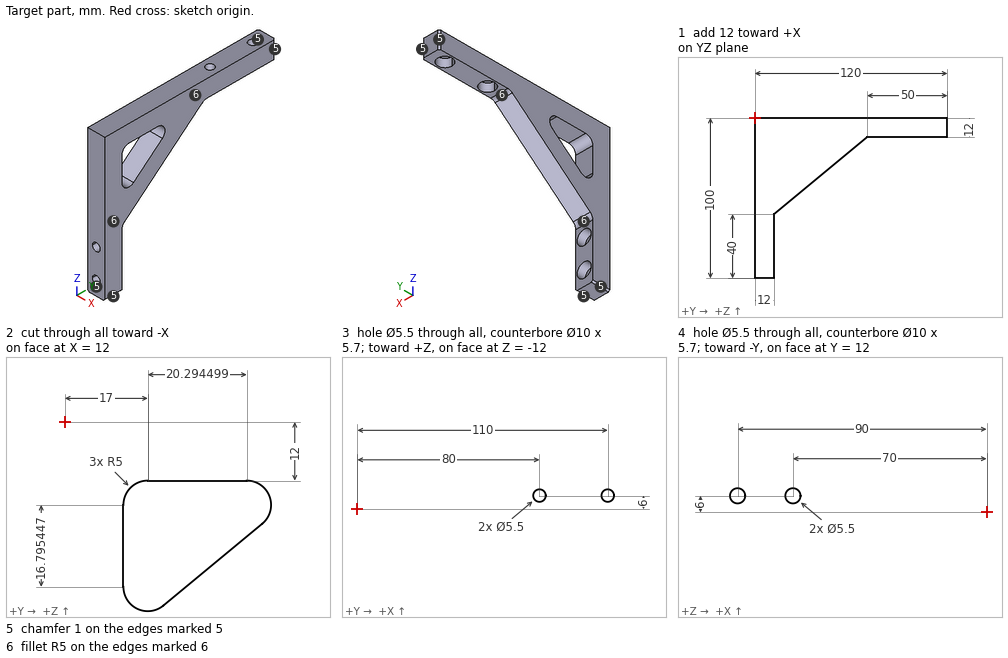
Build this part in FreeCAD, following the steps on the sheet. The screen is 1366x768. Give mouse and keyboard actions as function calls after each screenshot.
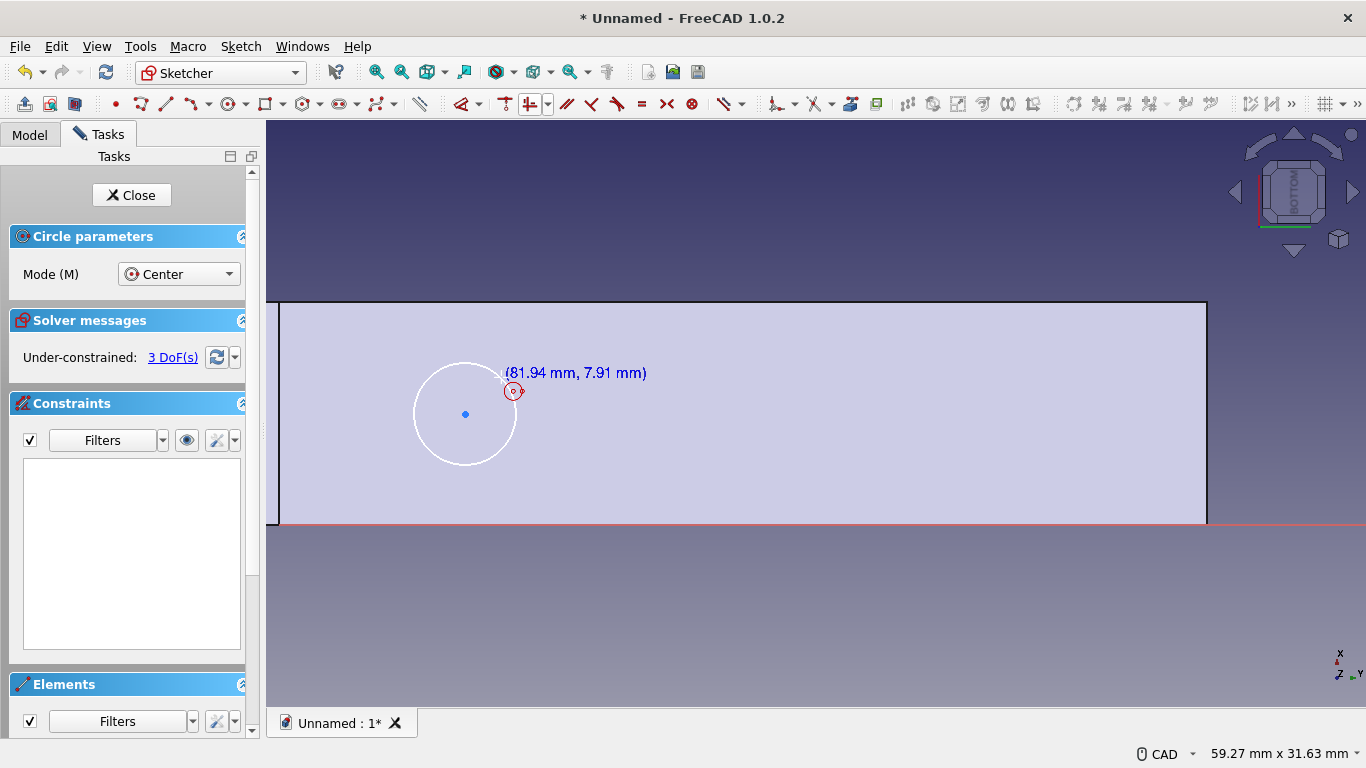
click(1022, 413)
click(1058, 377)
key(Escape)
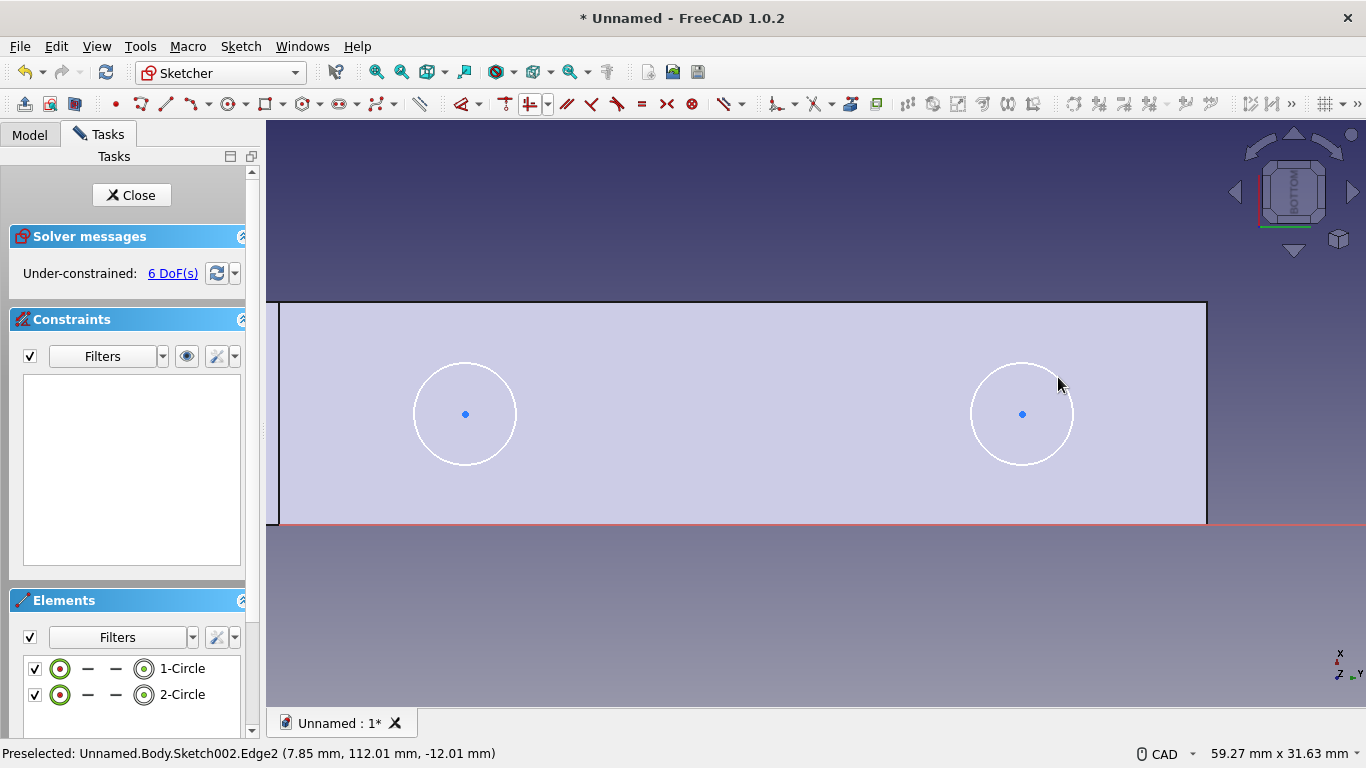
click(501, 378)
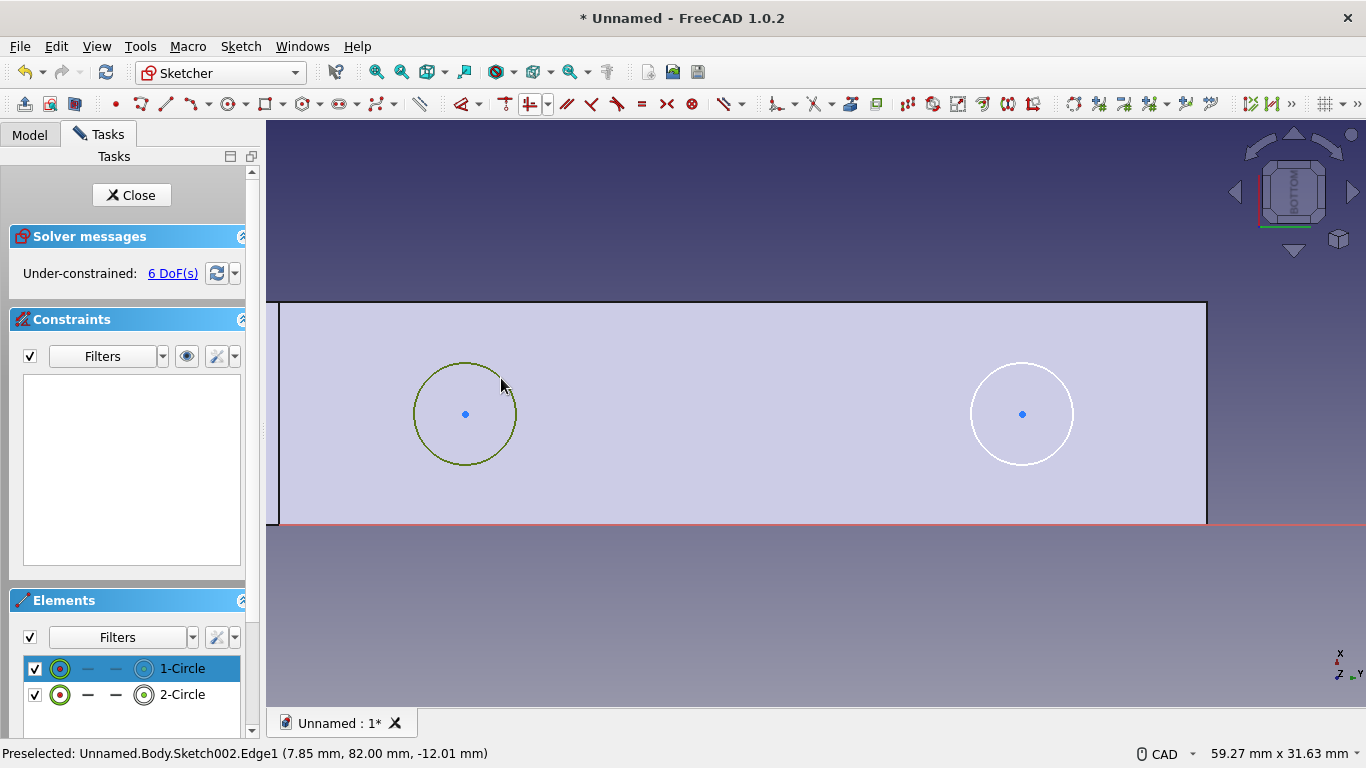
click(1058, 378)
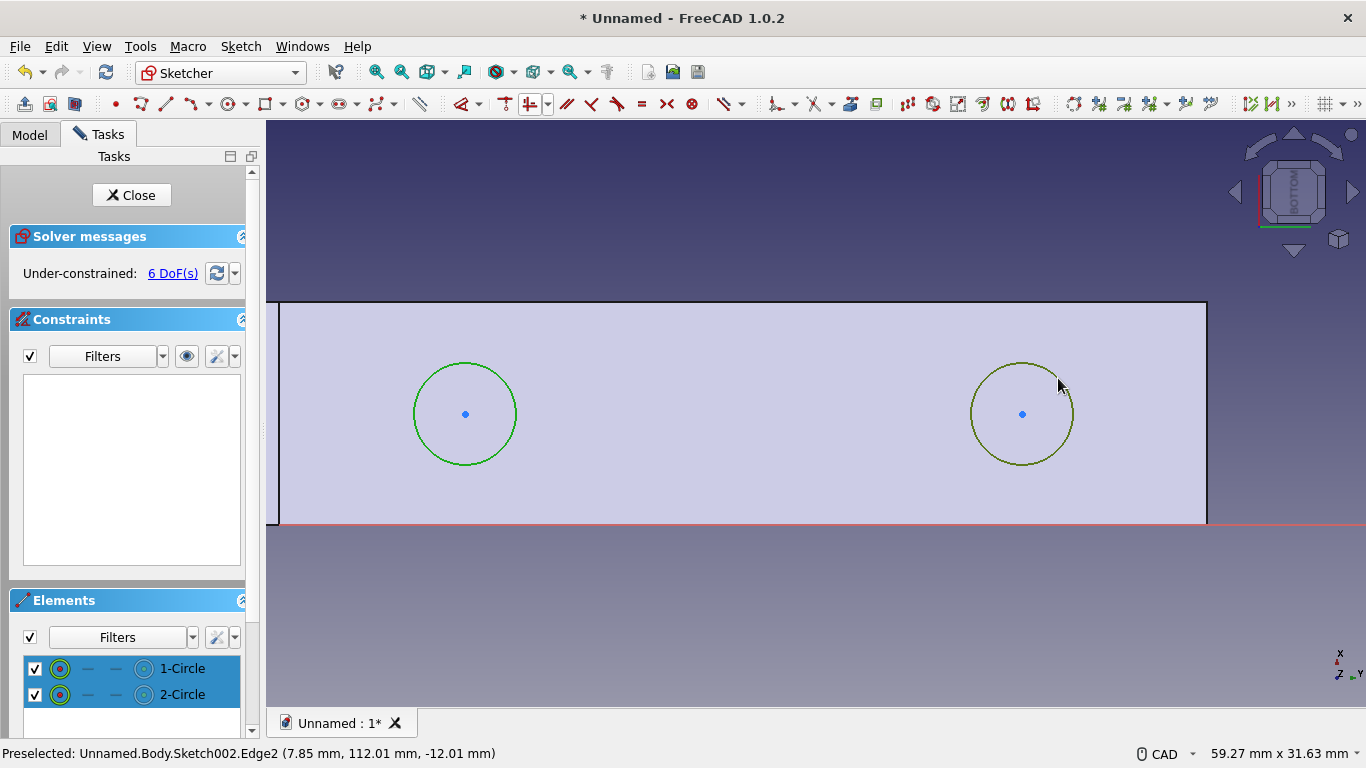
click(642, 104)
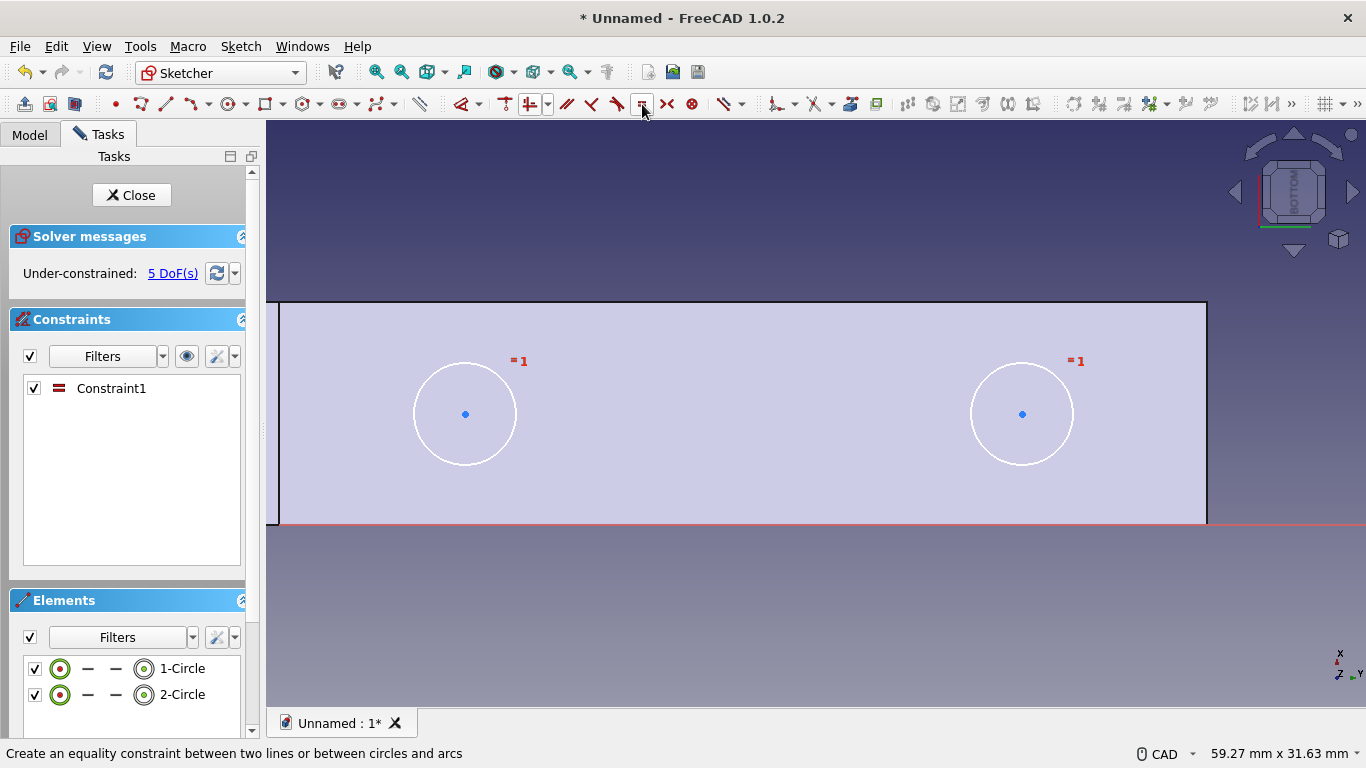
click(465, 414)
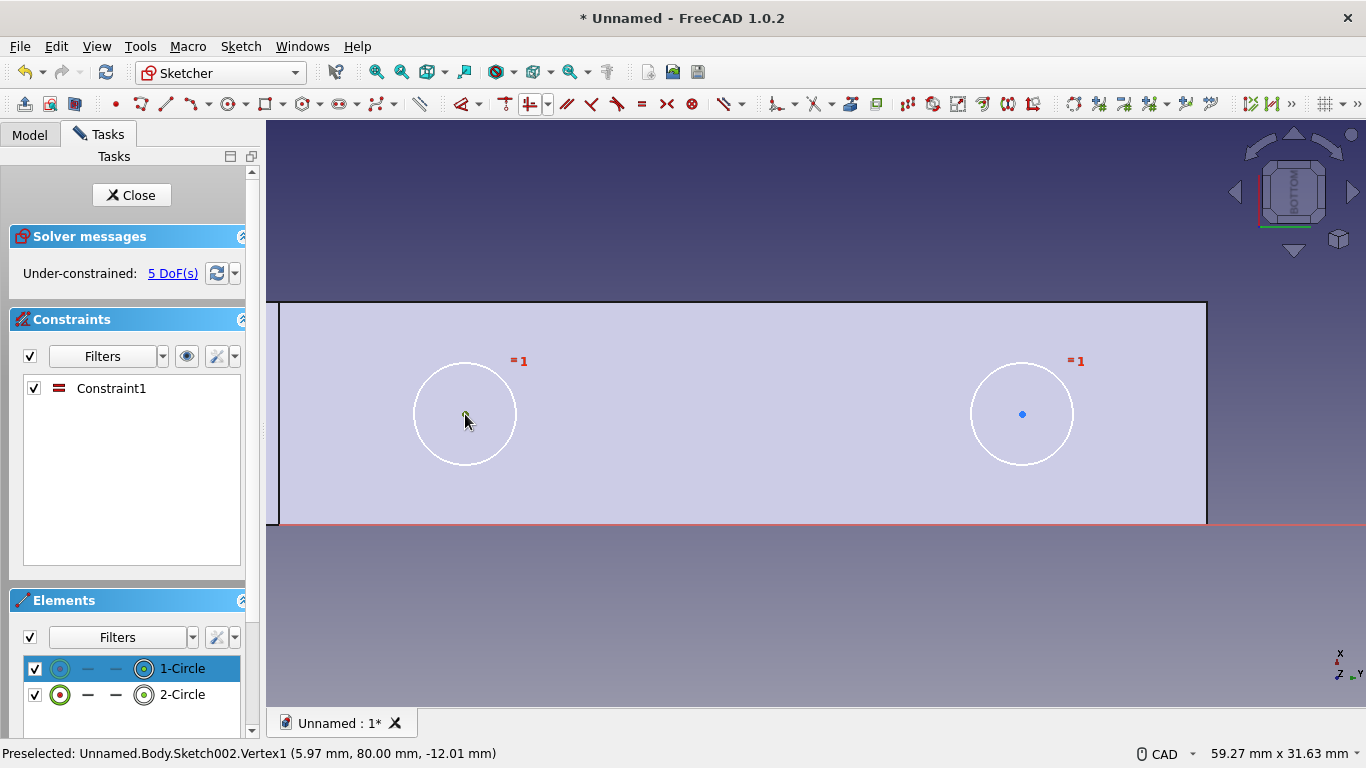
click(1022, 414)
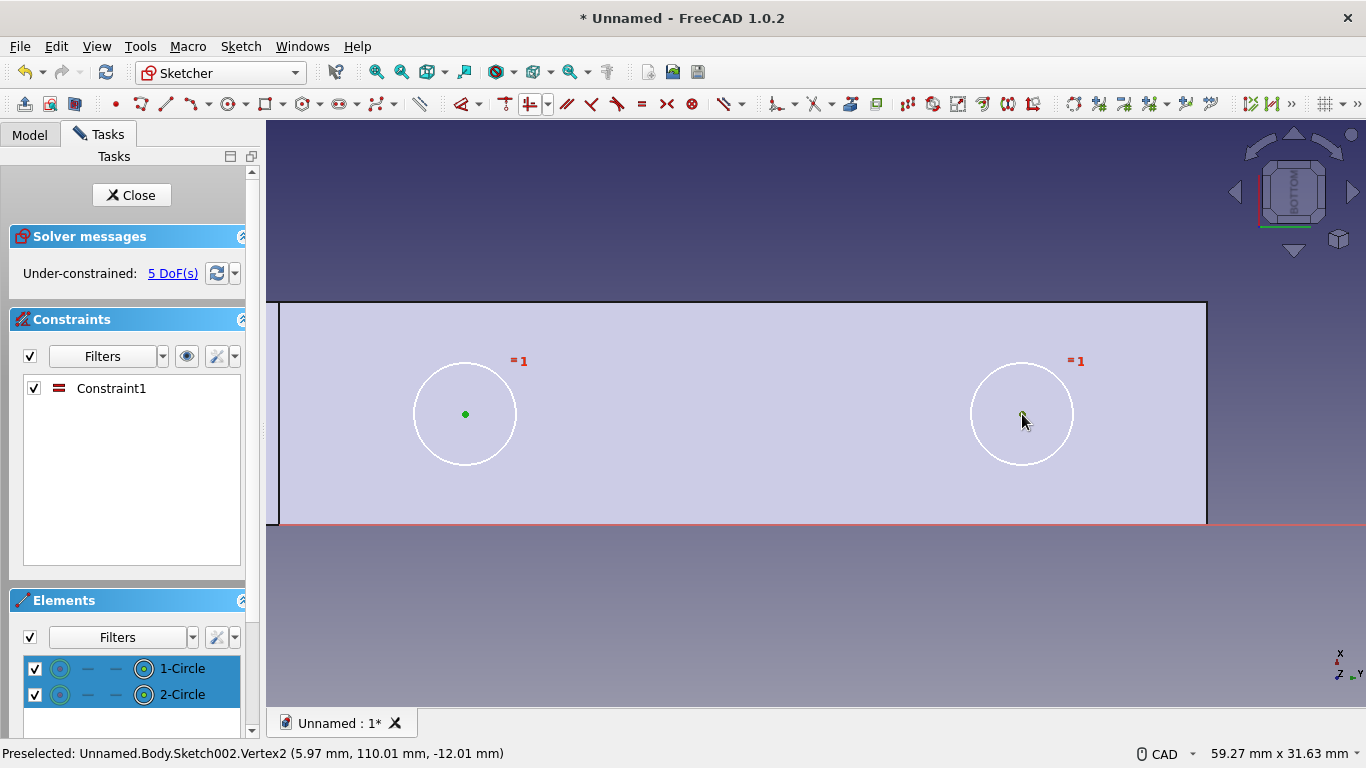
click(548, 104)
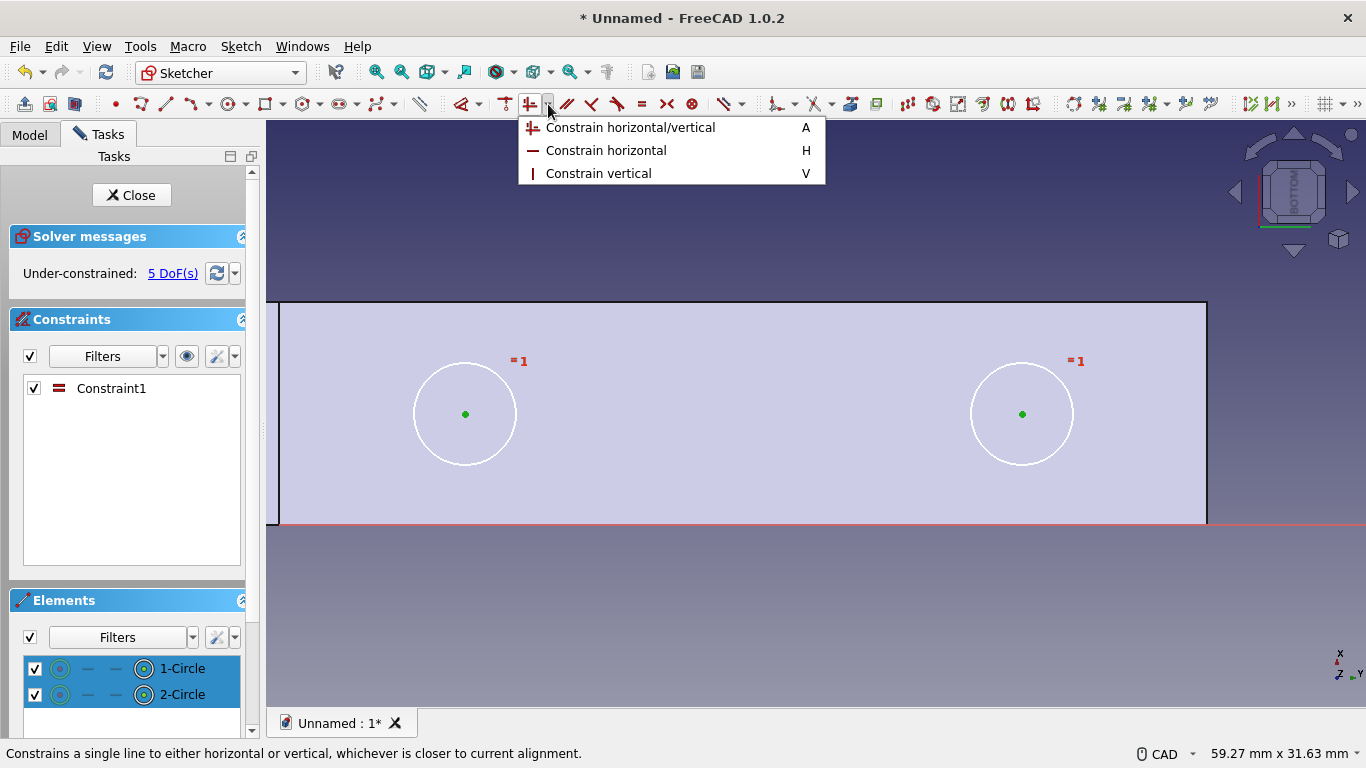
click(672, 150)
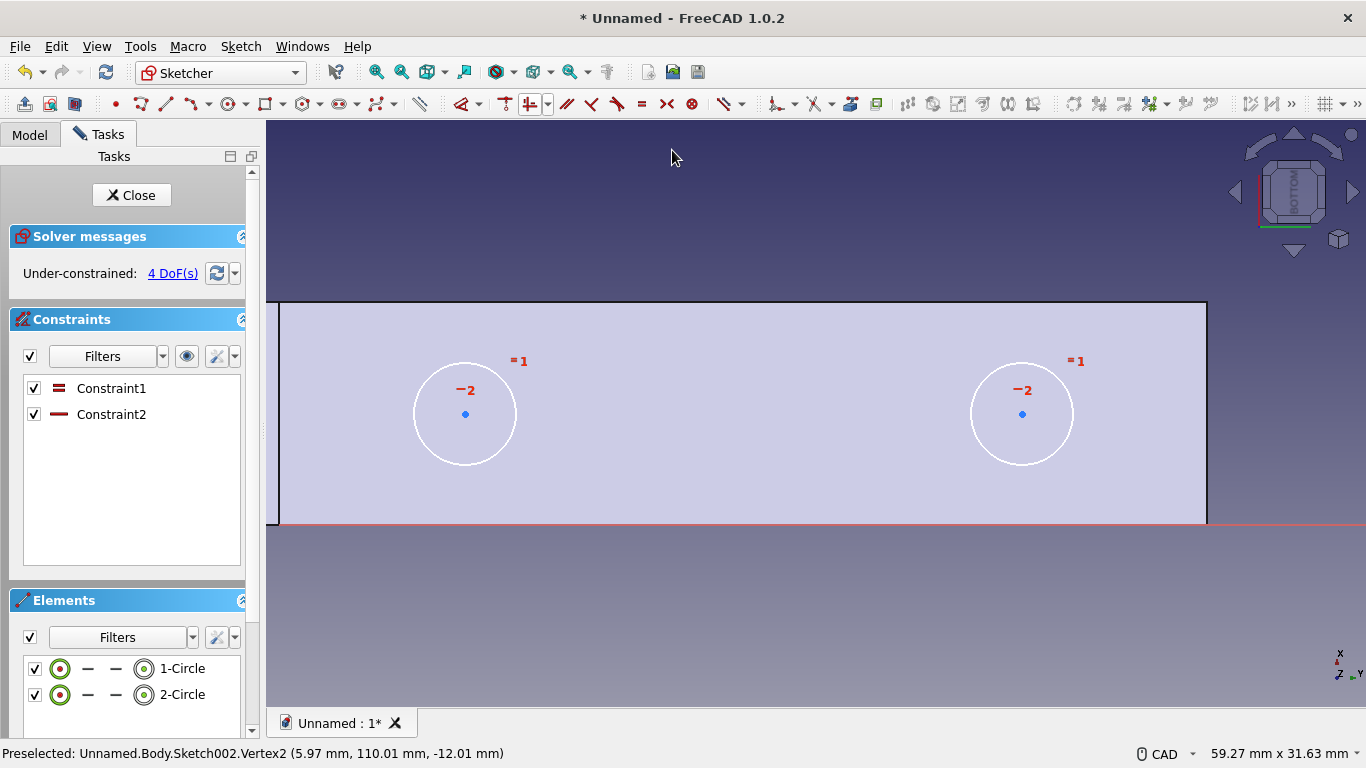
click(460, 104)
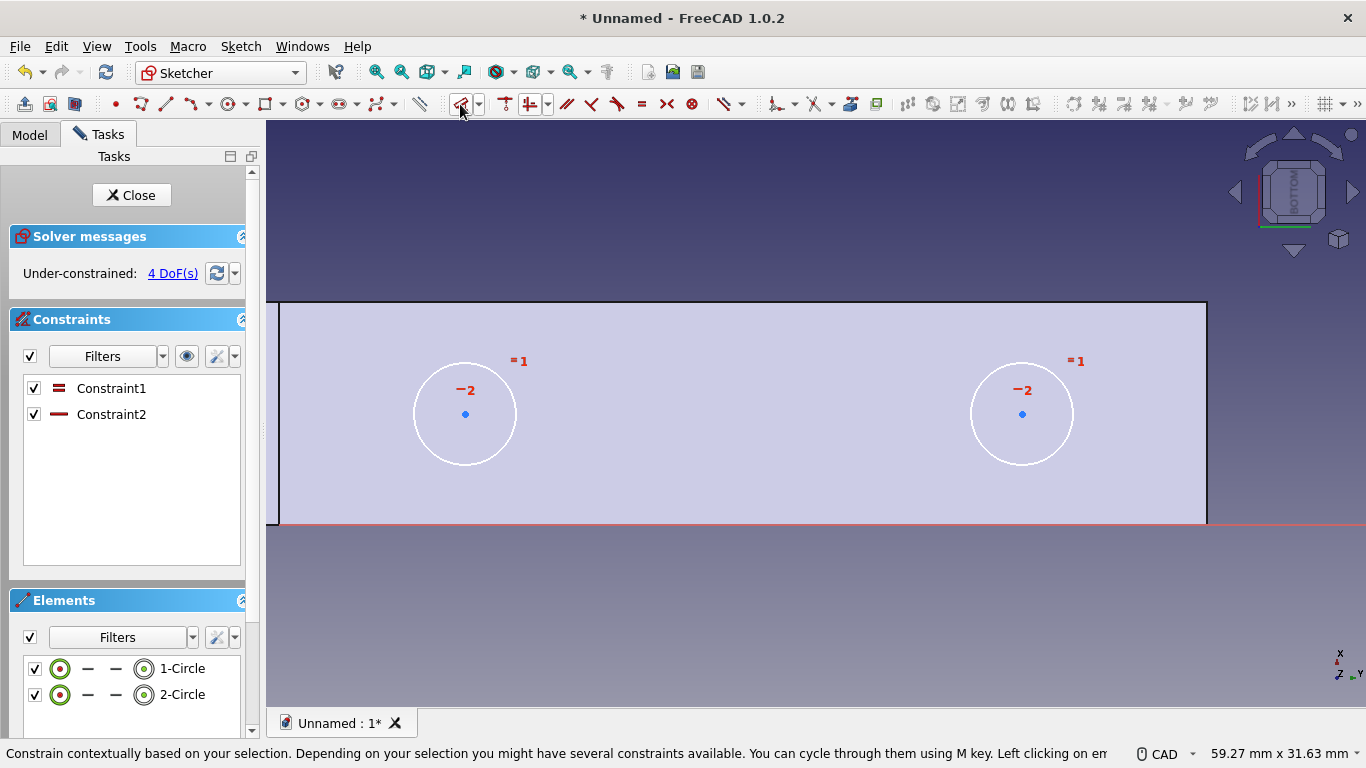
click(501, 378)
click(524, 355)